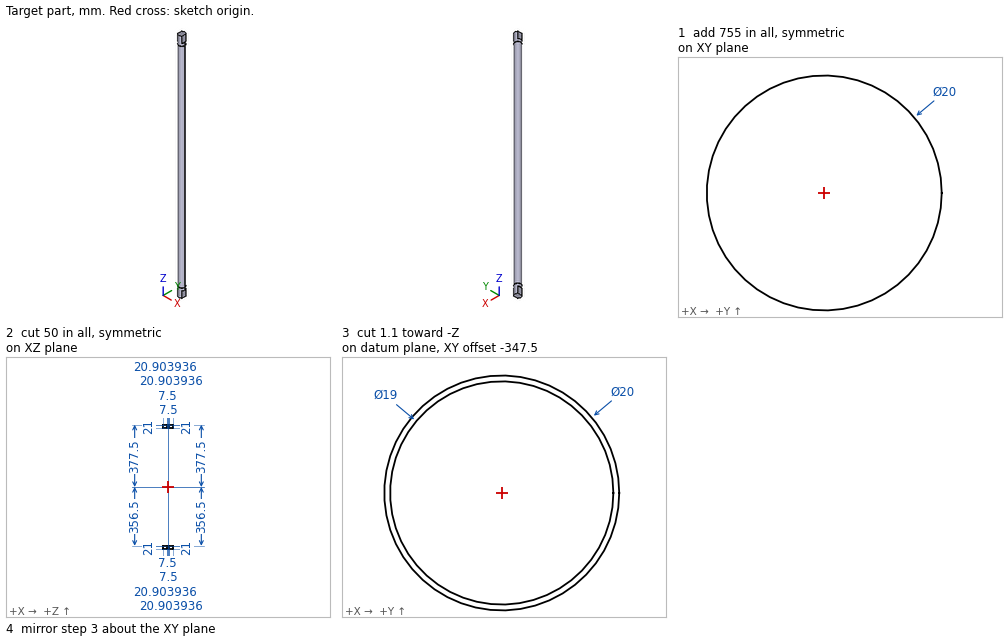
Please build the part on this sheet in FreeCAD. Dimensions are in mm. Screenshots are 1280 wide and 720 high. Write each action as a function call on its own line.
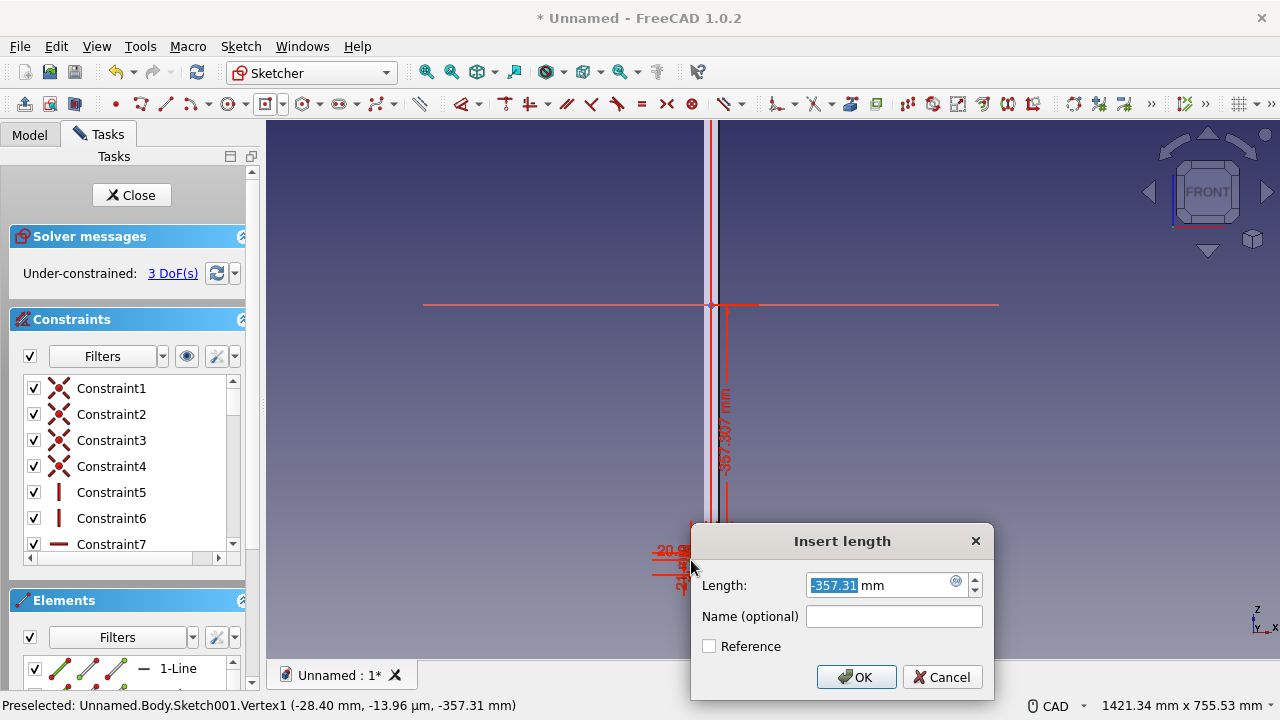
text(-356.5)
key(Return)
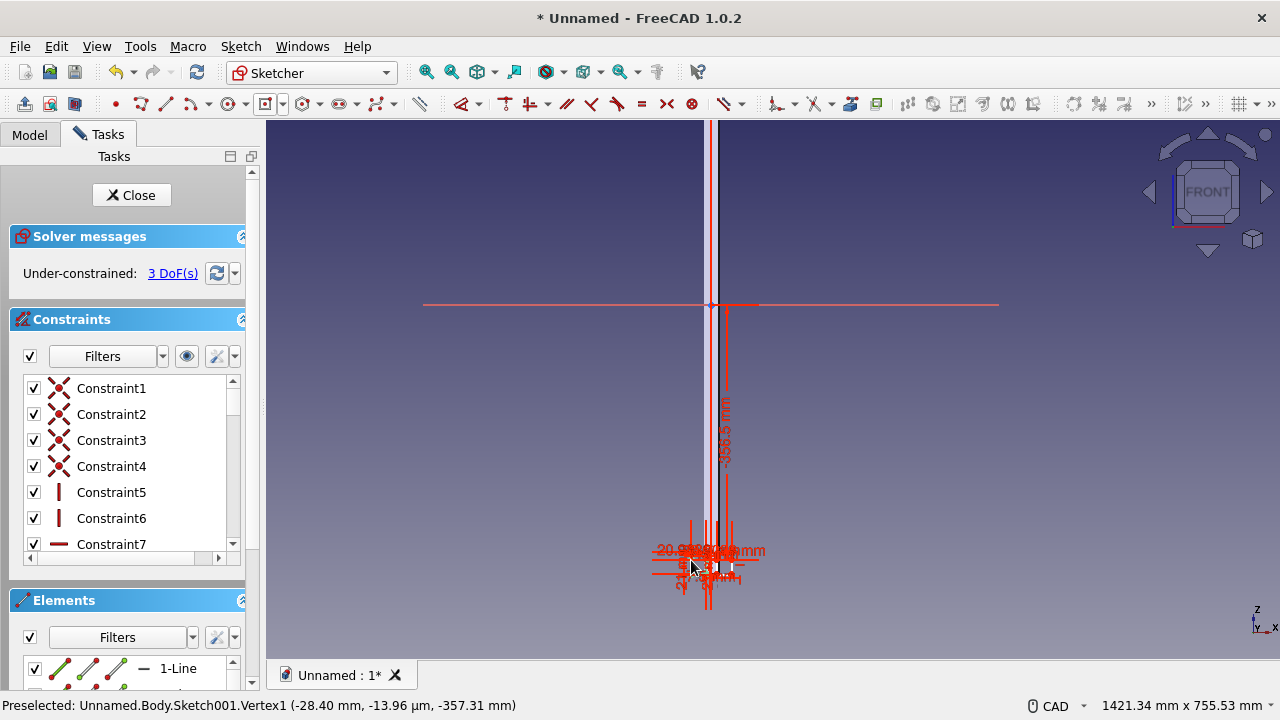
click(717, 560)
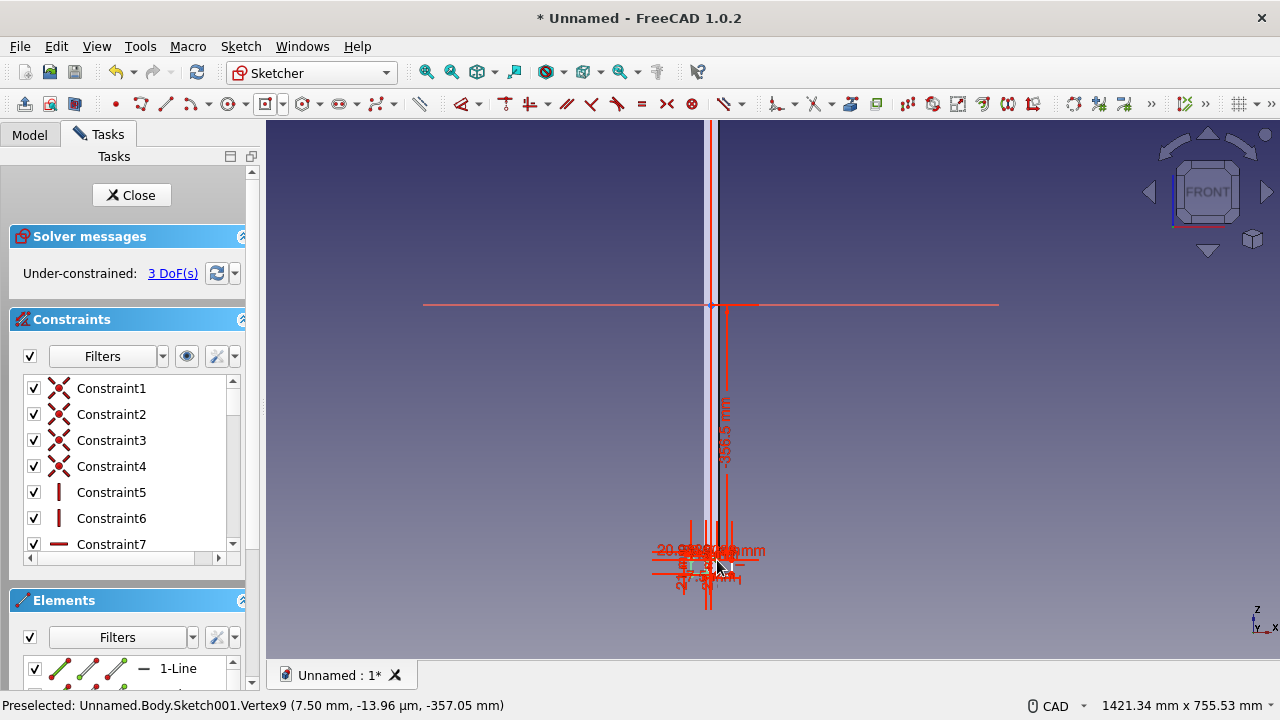
key(i)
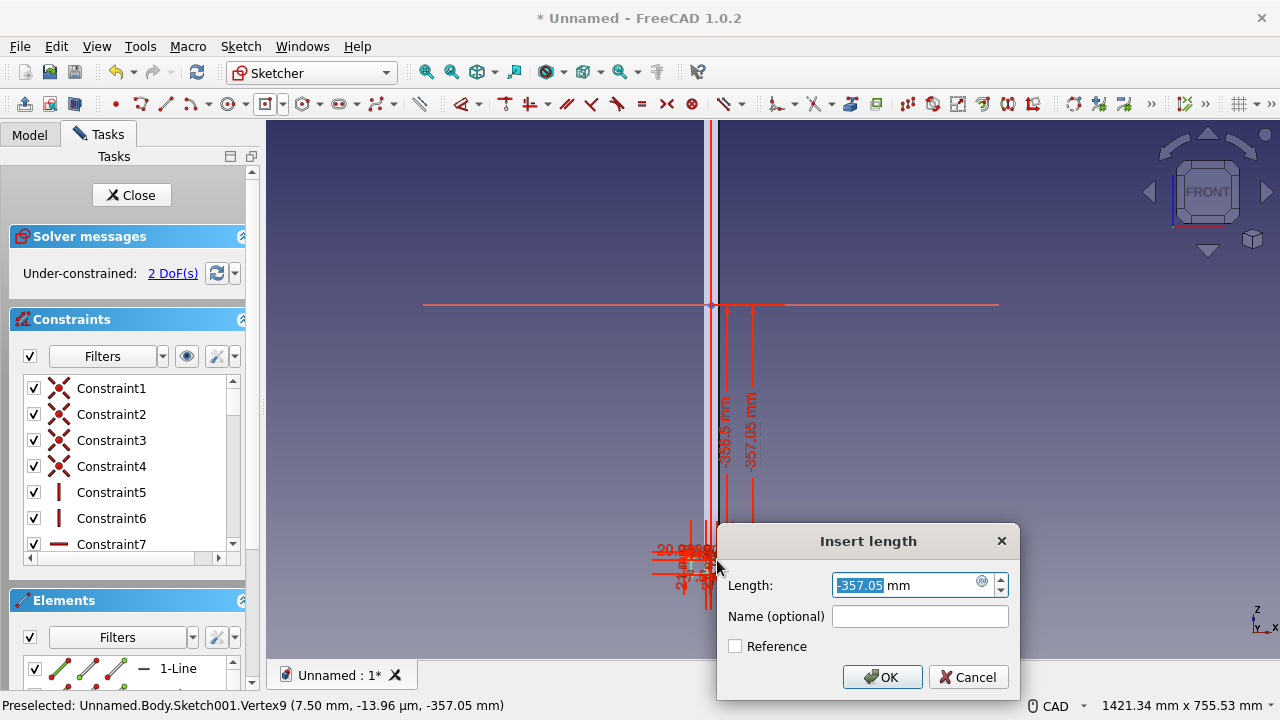
text(-356.5)
key(Return)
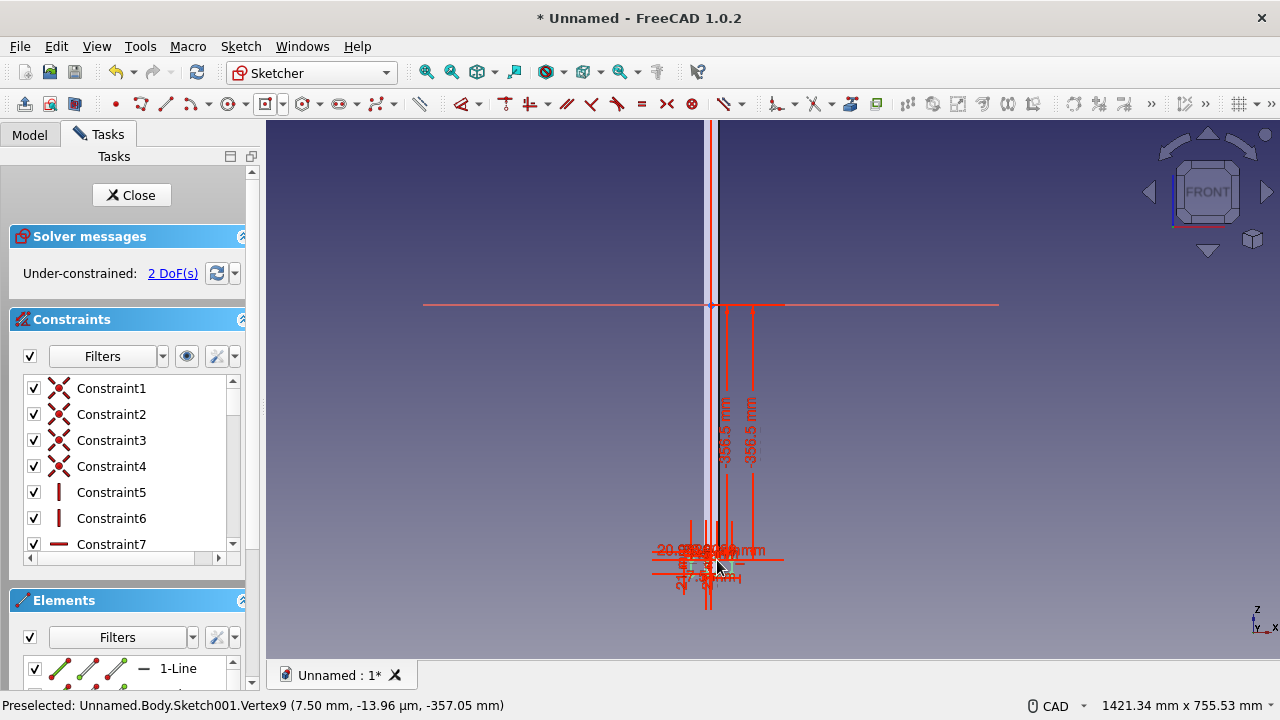
scroll(690, 561, down, 2)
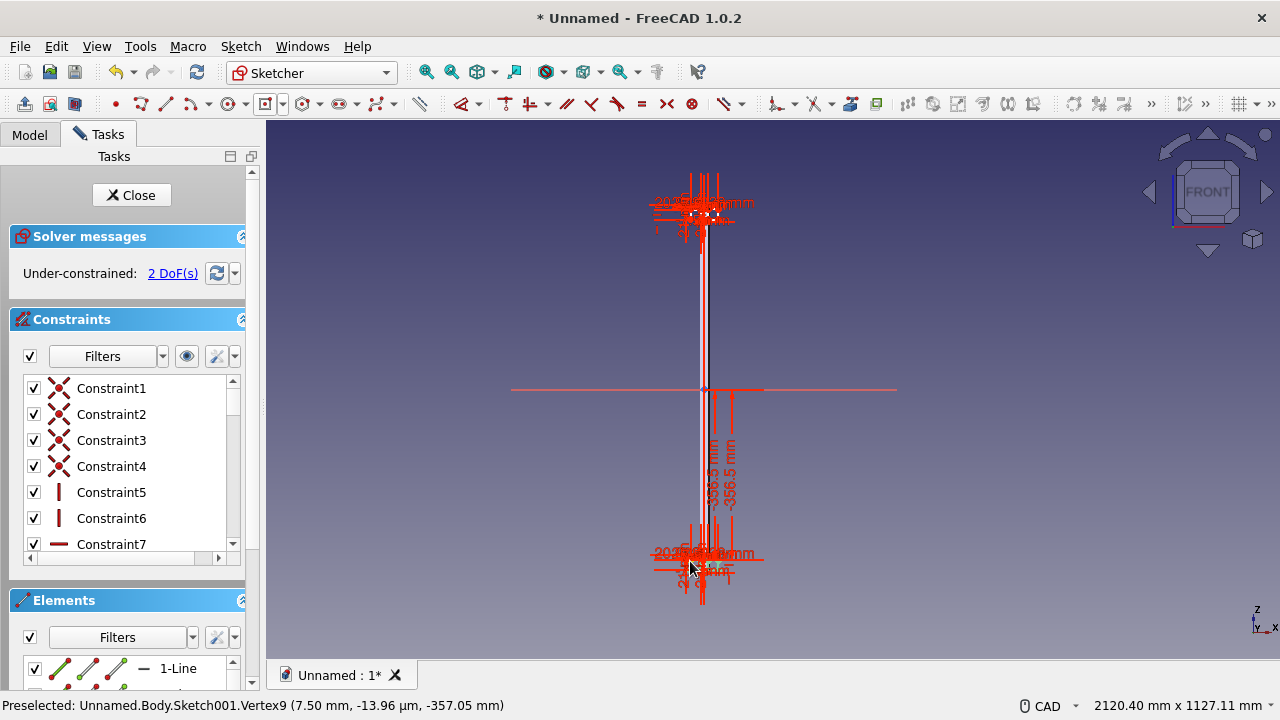
scroll(708, 209, up, 3)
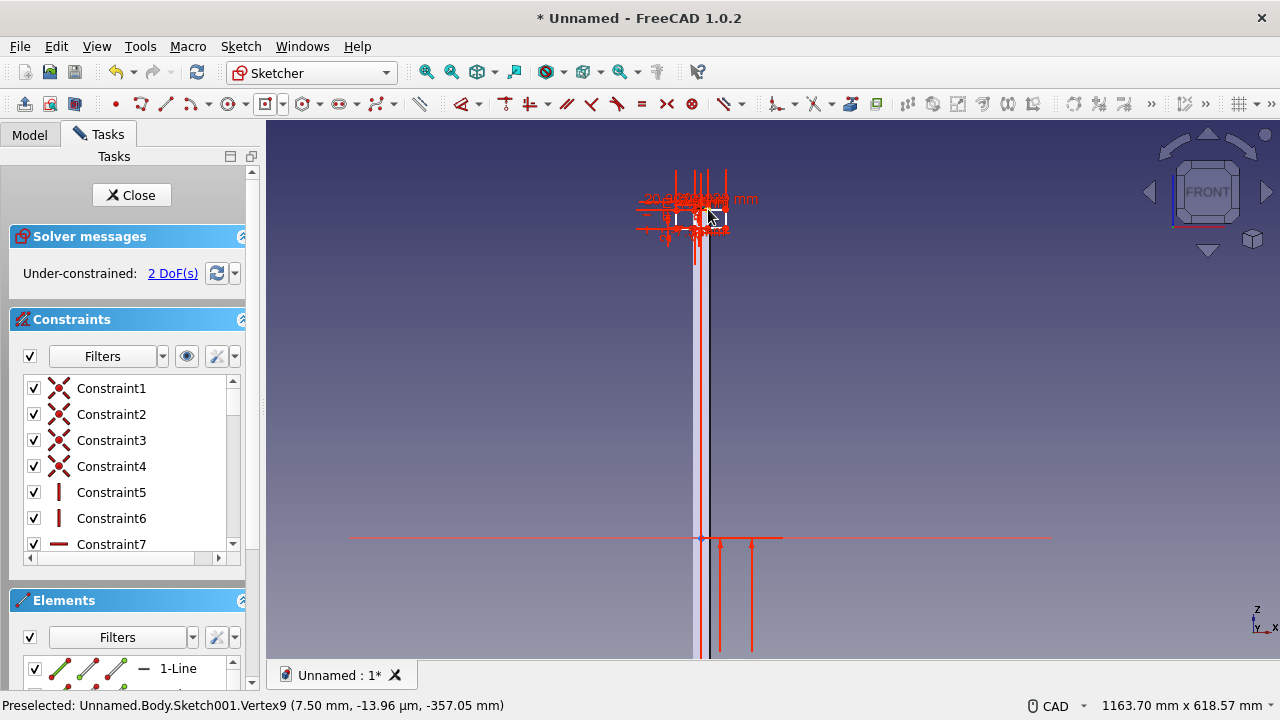
click(708, 210)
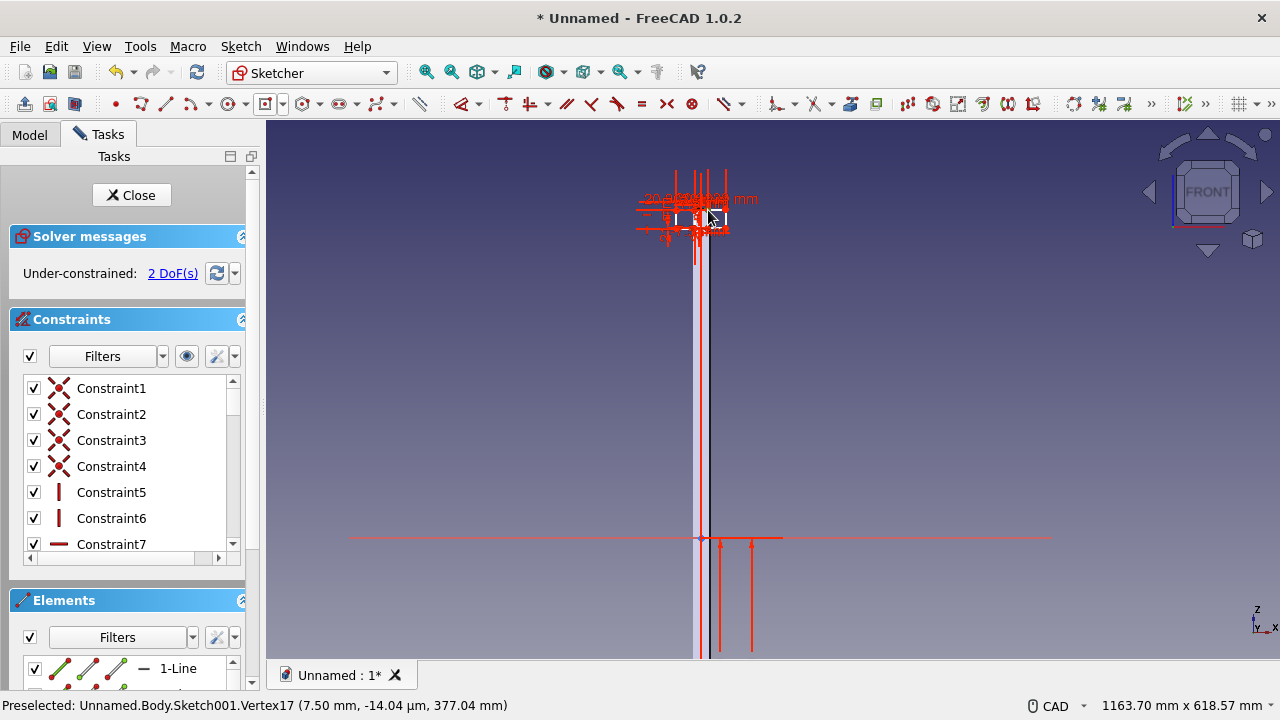
key(i)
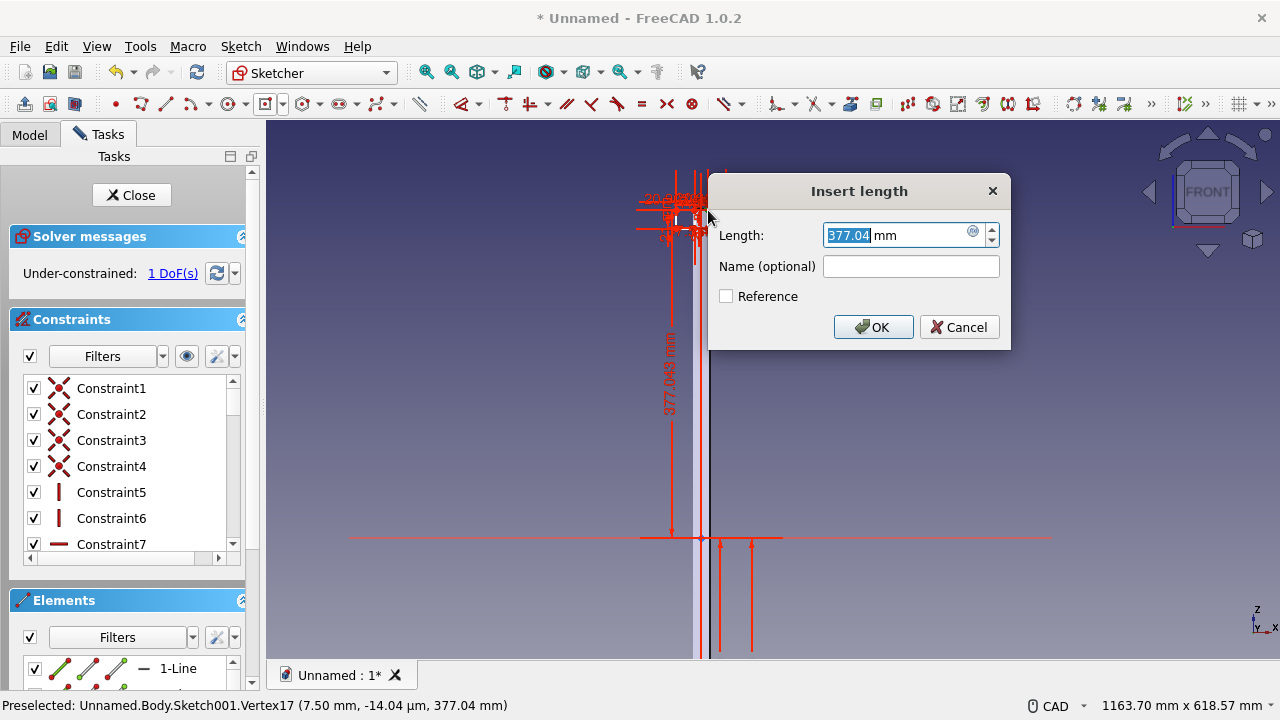
text(377.5)
key(Return)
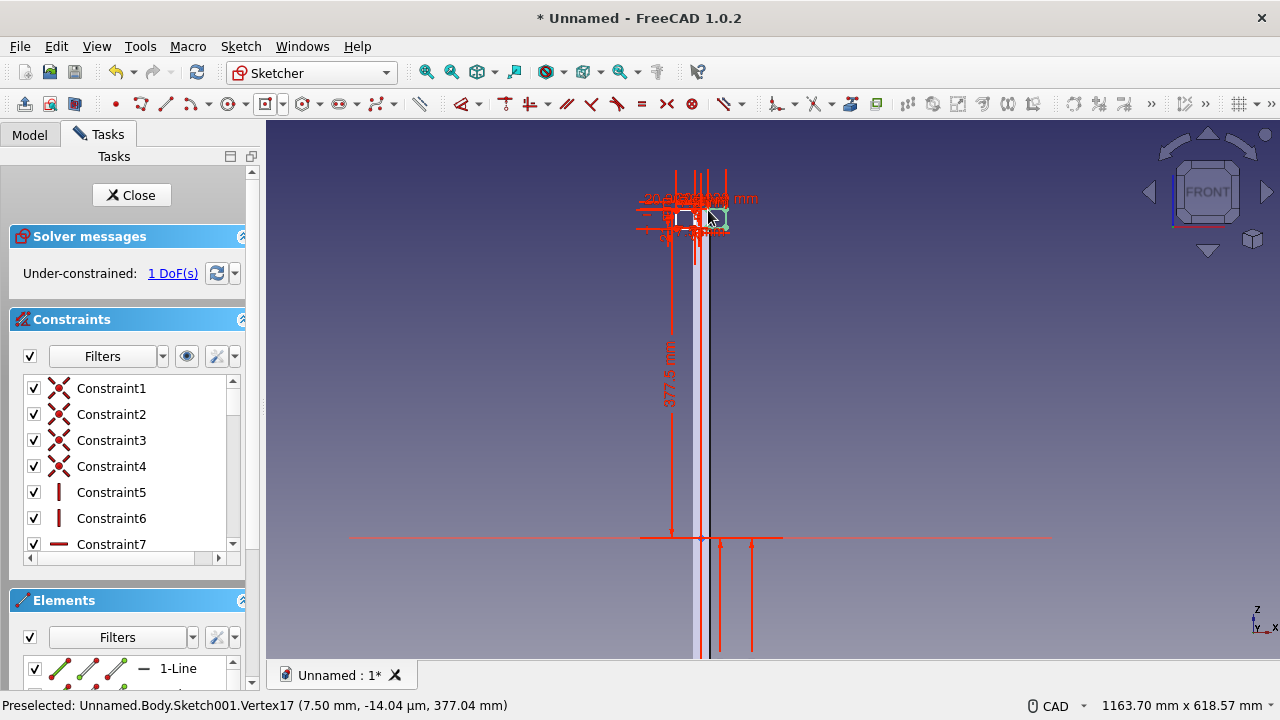
click(676, 210)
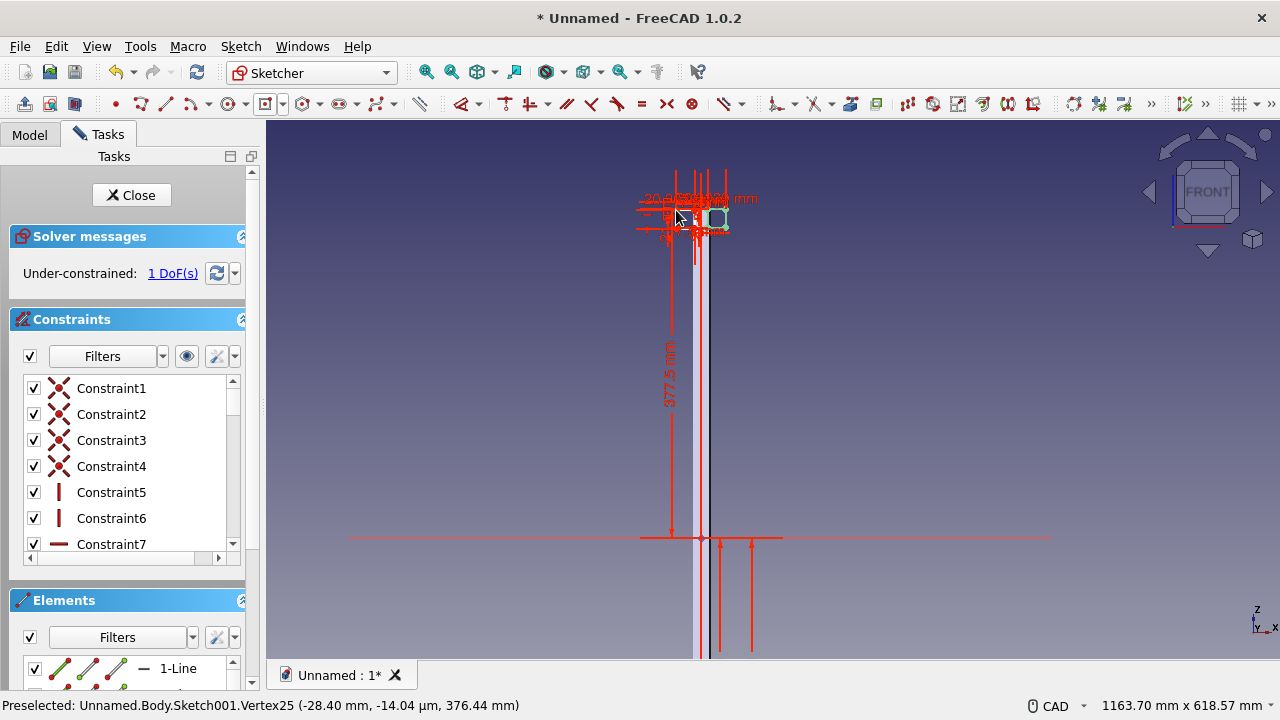
key(i)